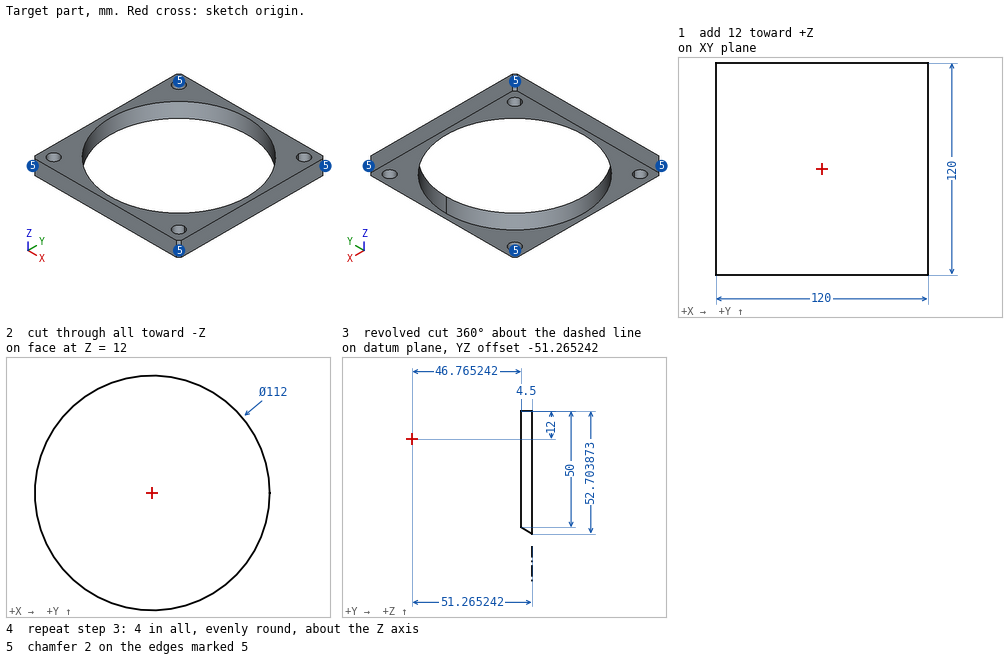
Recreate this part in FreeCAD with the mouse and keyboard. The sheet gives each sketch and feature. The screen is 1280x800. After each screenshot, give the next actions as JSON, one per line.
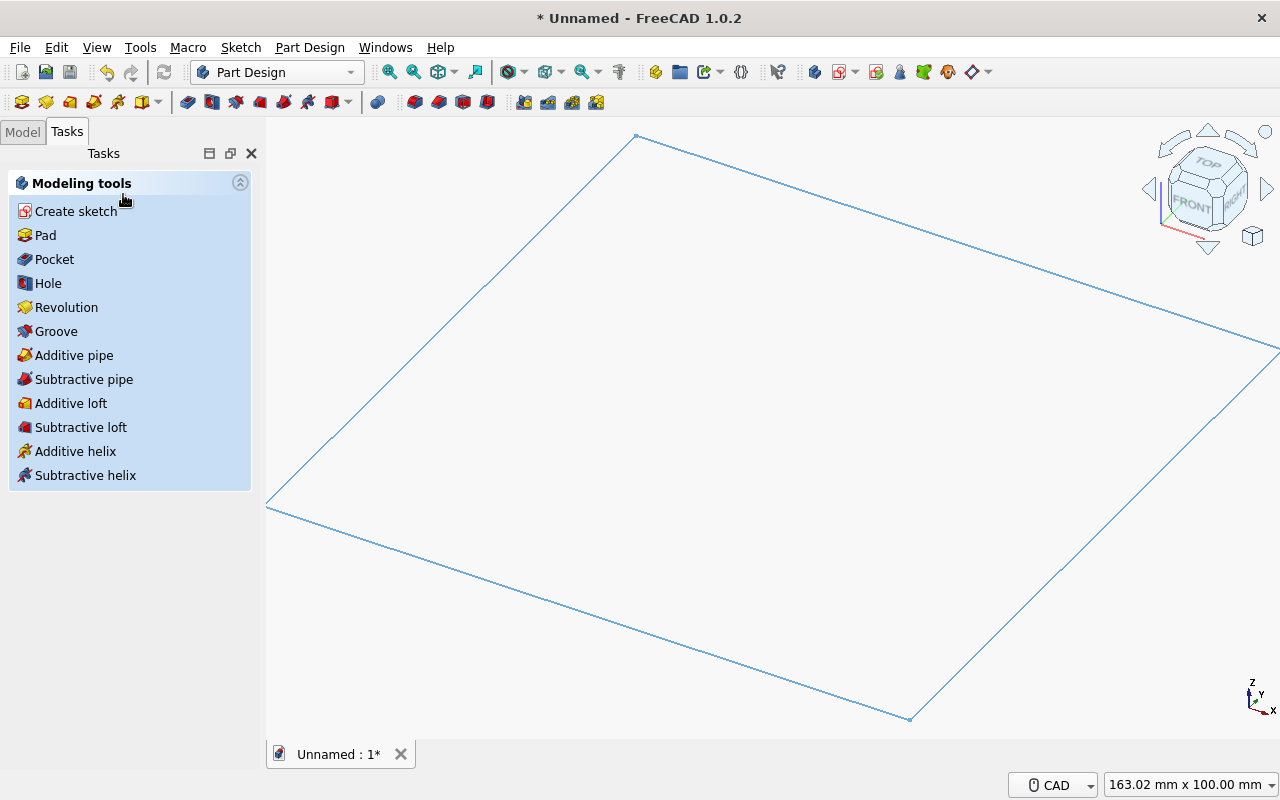
{"action": "left_click", "coordinate": [22, 102]}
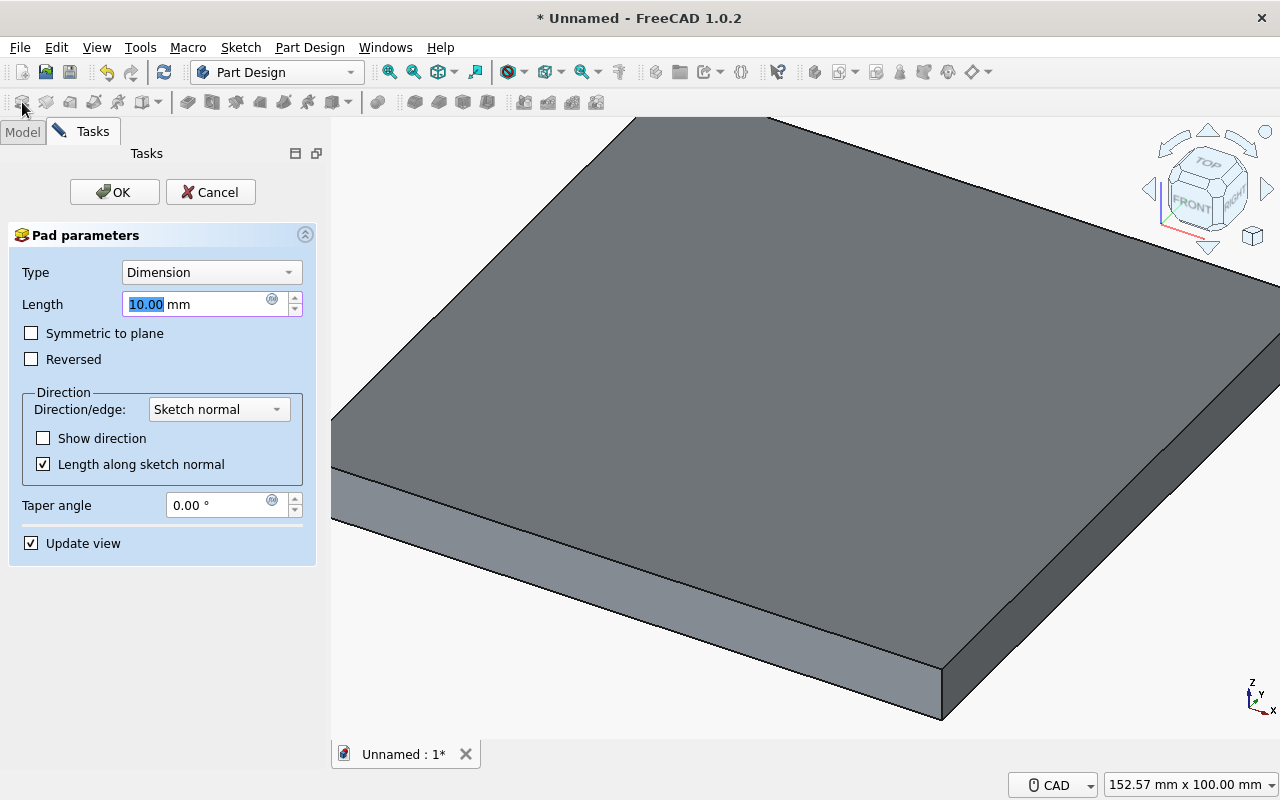
{"action": "type", "text": "12"}
{"action": "key", "text": "Tab"}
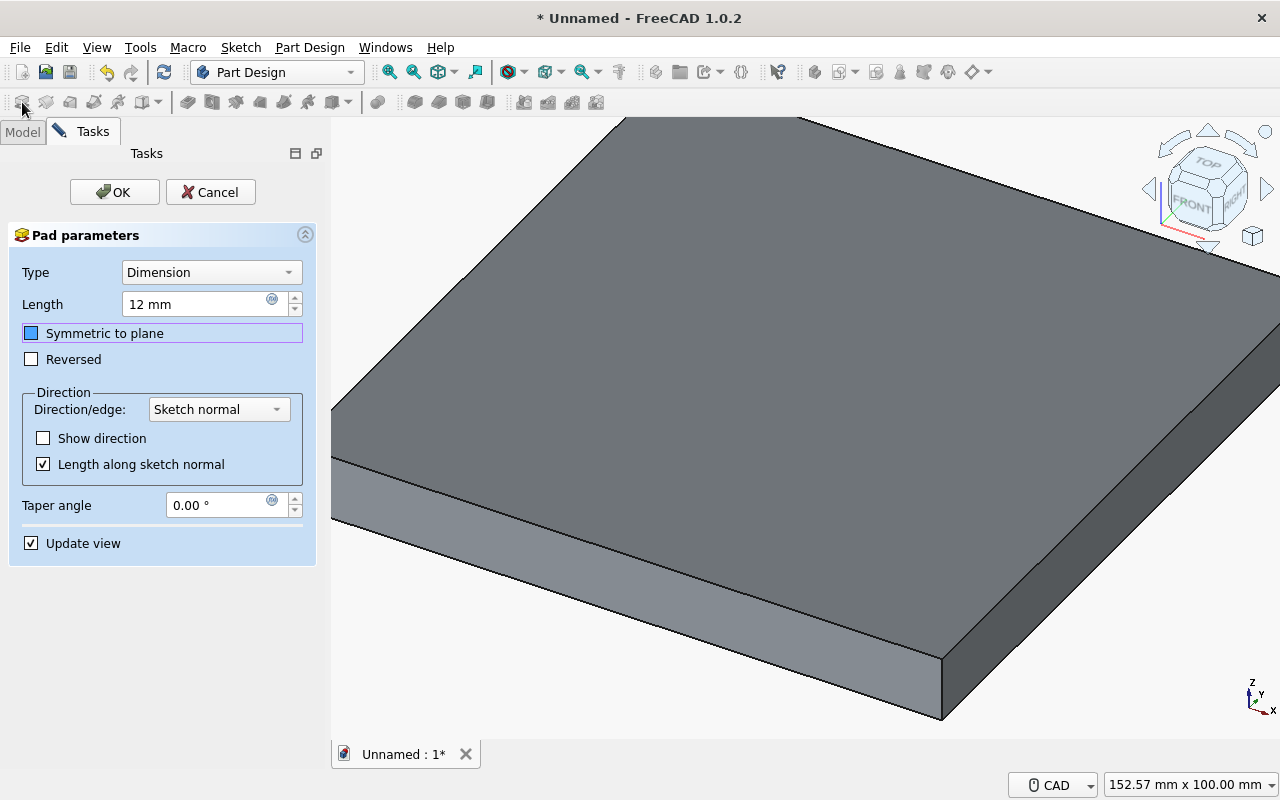
{"action": "left_click", "coordinate": [115, 192]}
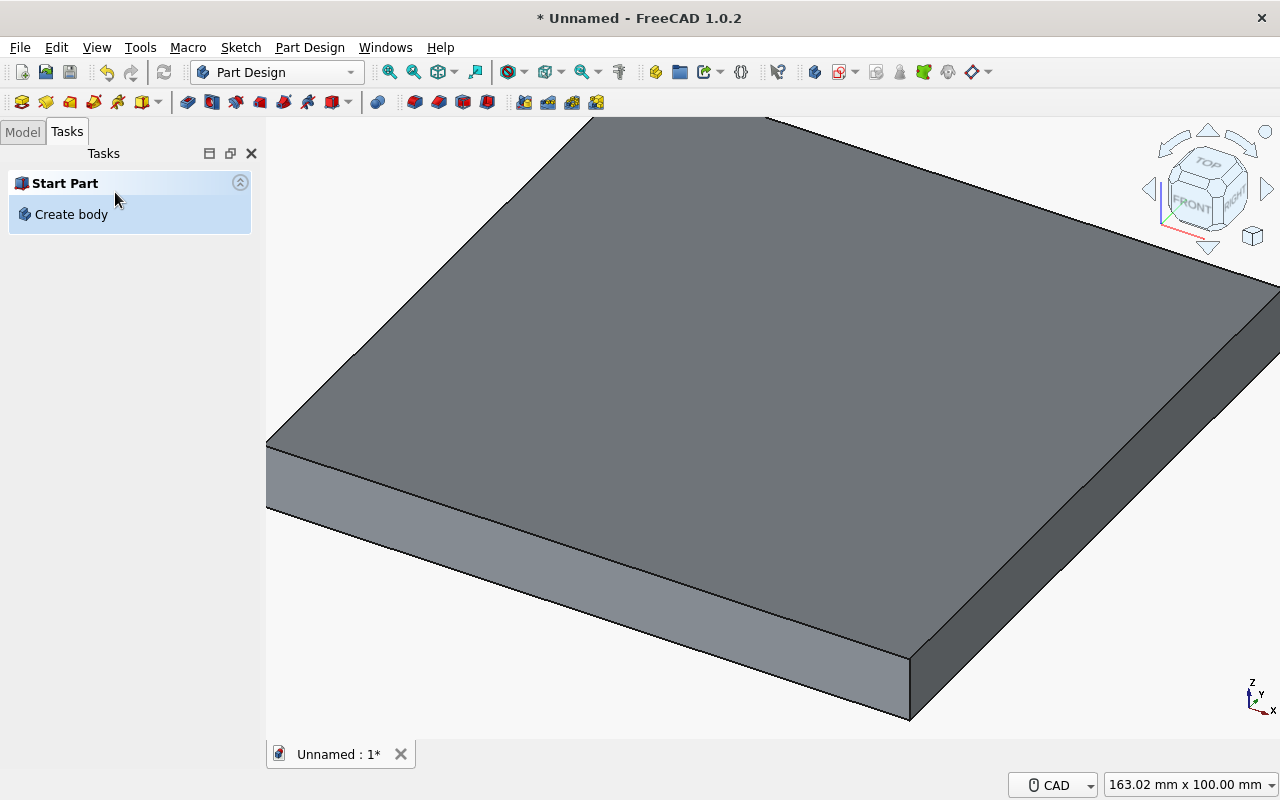
{"action": "left_click", "coordinate": [390, 72]}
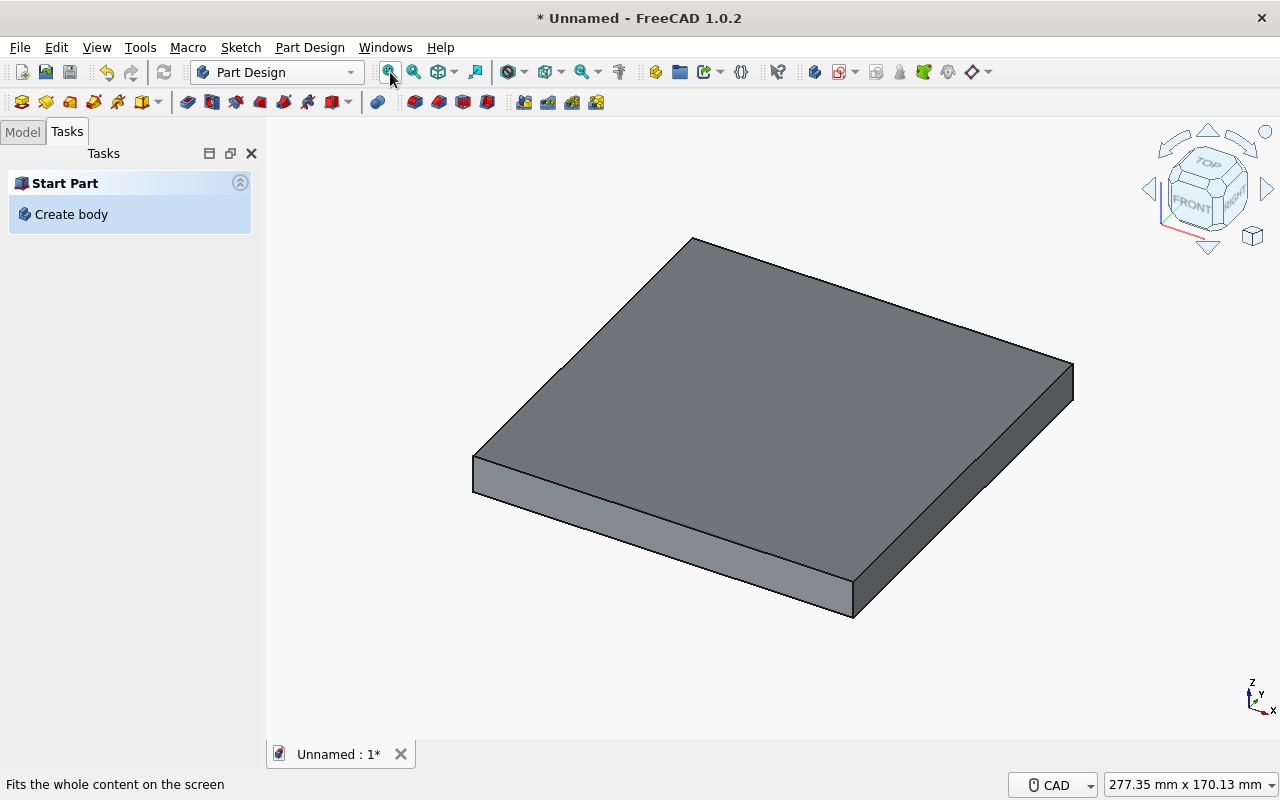
{"action": "left_click", "coordinate": [773, 409]}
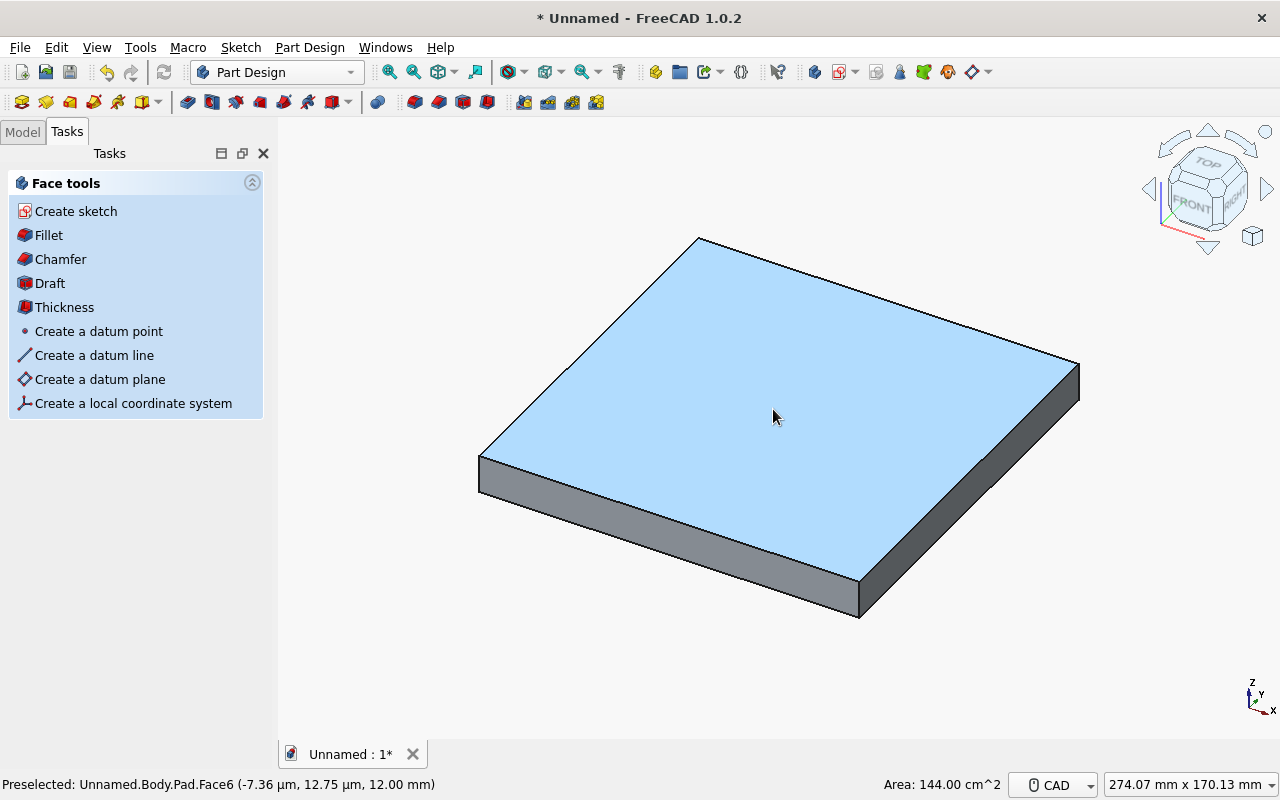
{"action": "left_click", "coordinate": [840, 72]}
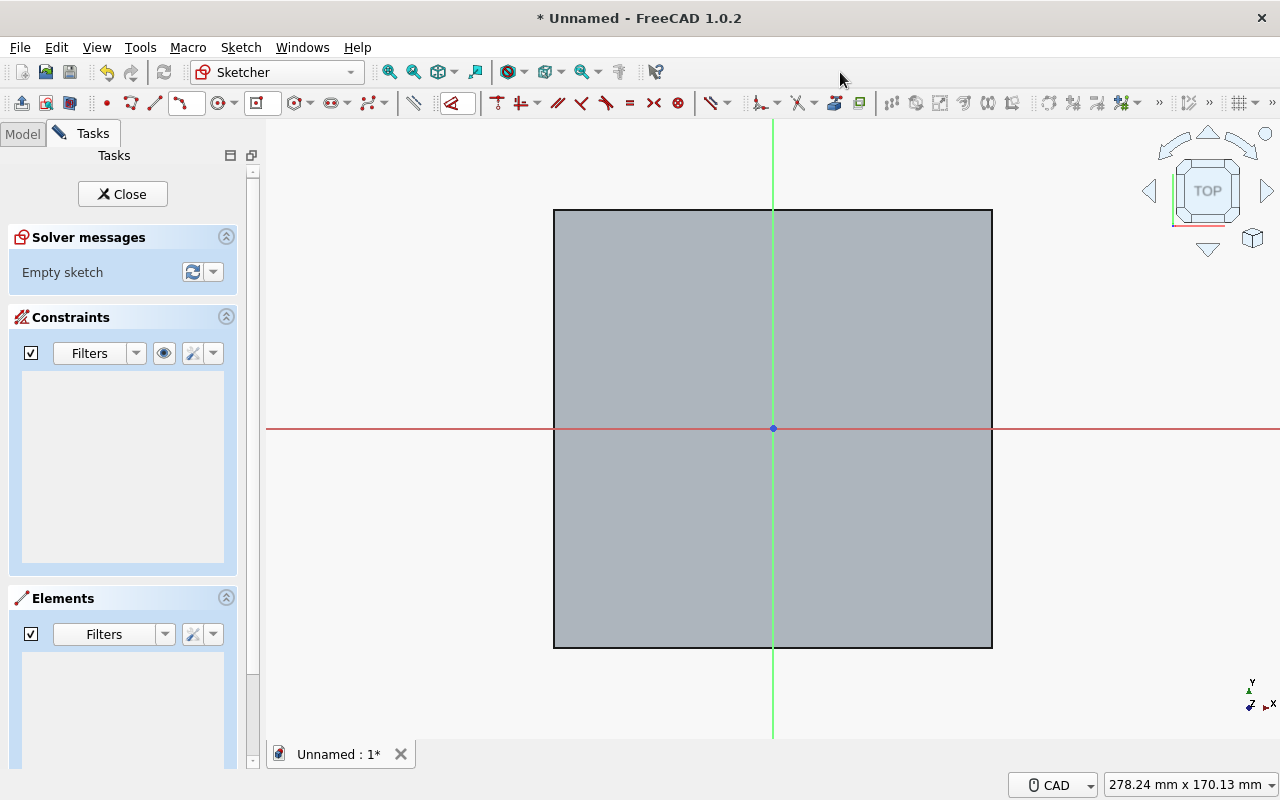
{"action": "left_click", "coordinate": [218, 104]}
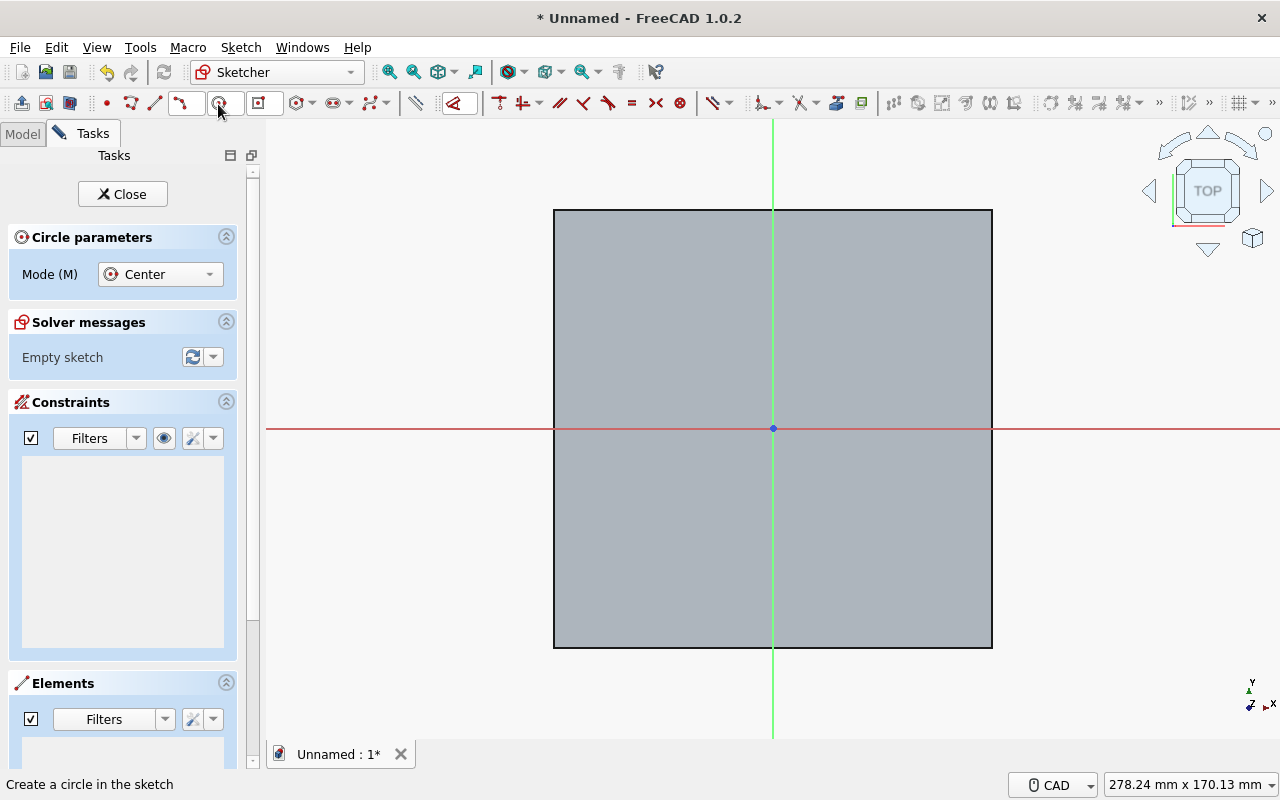
{"action": "left_click", "coordinate": [773, 429]}
{"action": "mouse_move", "coordinate": [917, 285]}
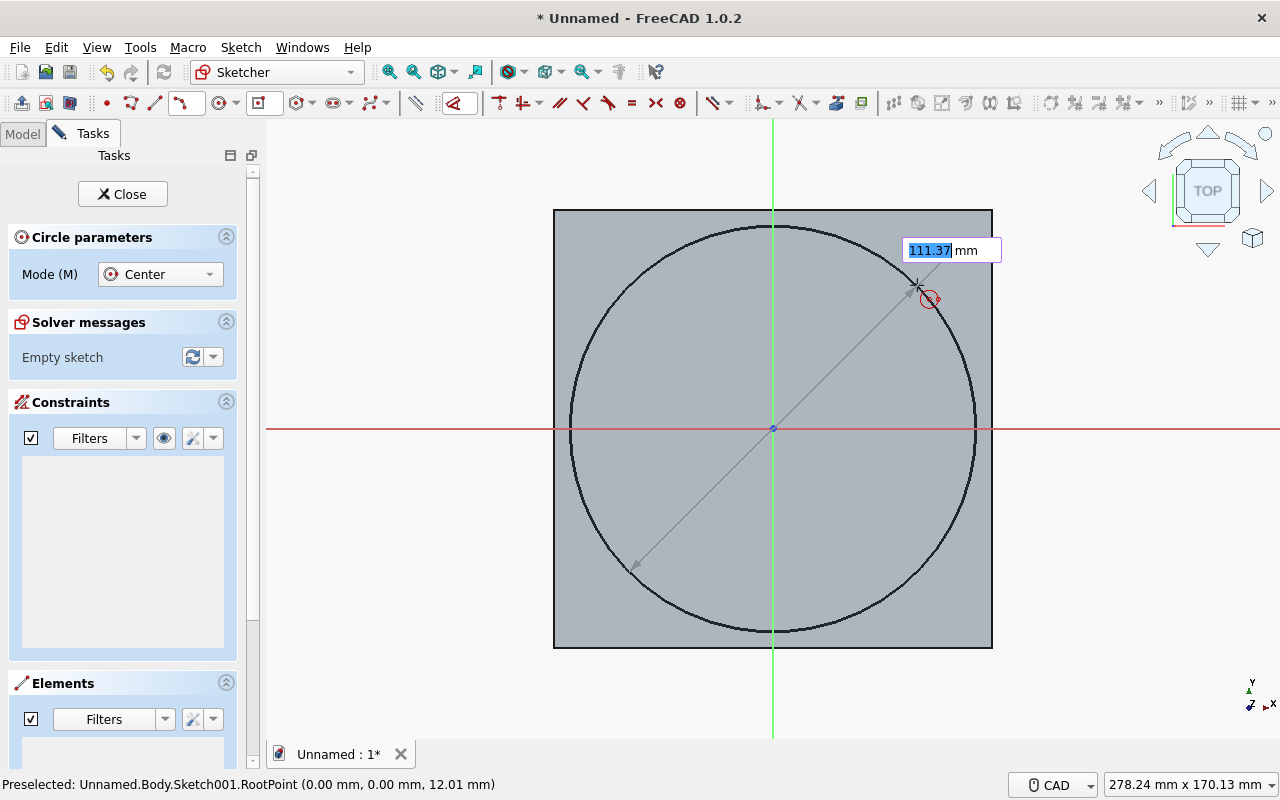
{"action": "type", "text": "112"}
{"action": "key", "text": "Return"}
{"action": "key", "text": "Escape"}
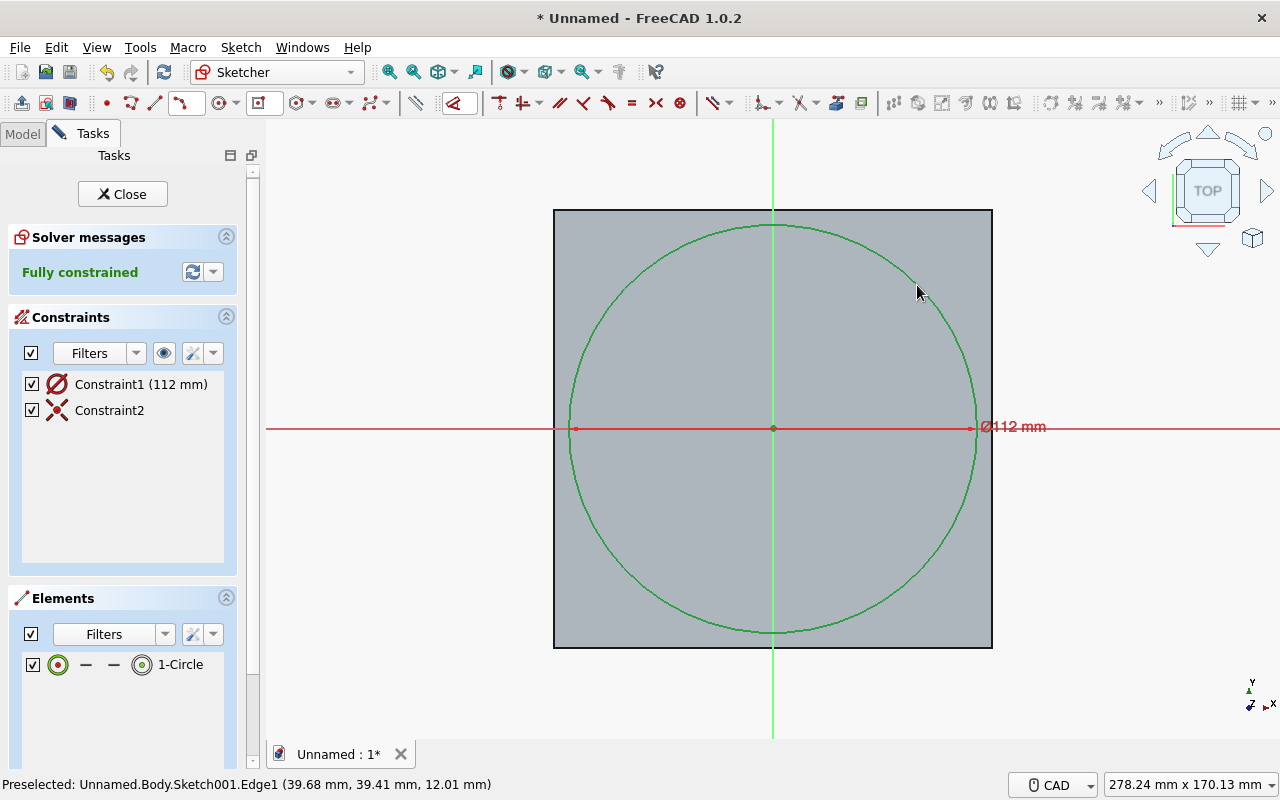
{"action": "left_click", "coordinate": [123, 194]}